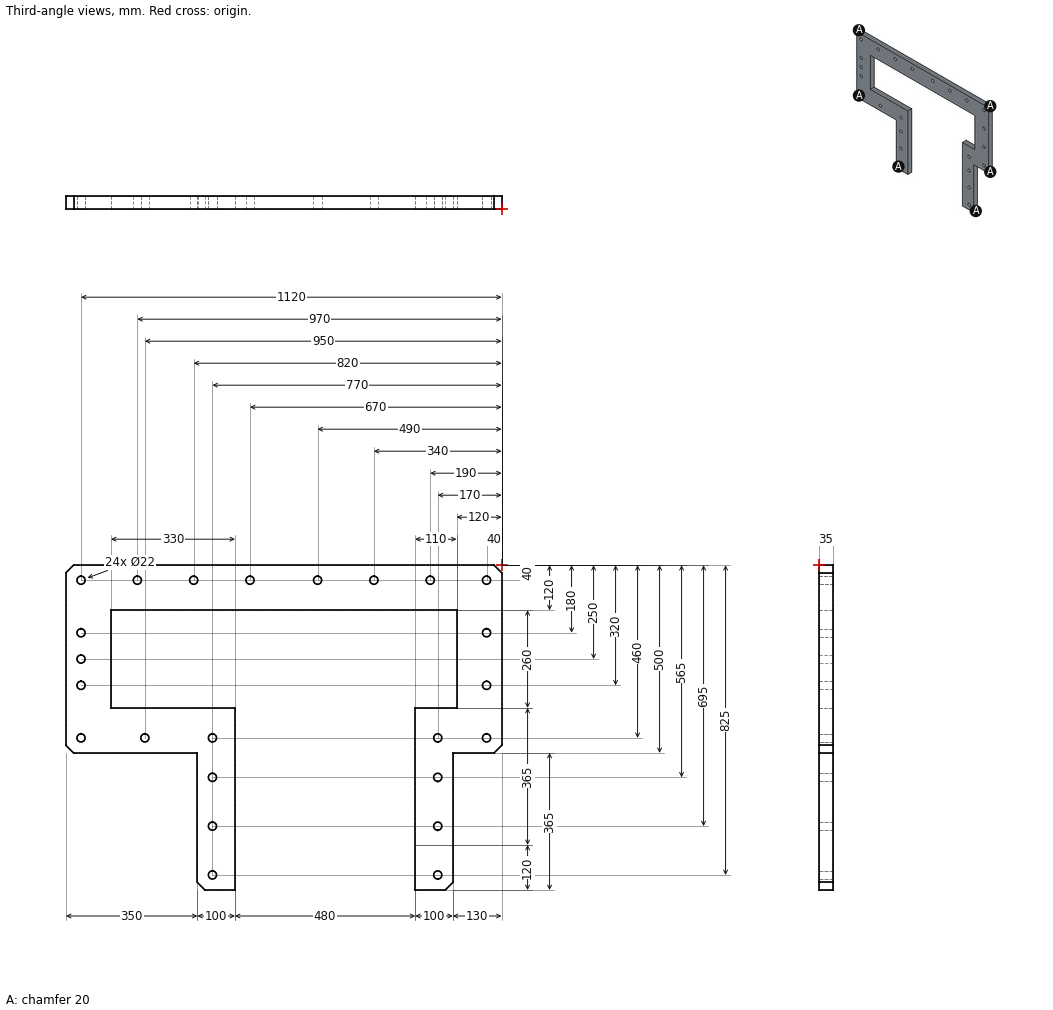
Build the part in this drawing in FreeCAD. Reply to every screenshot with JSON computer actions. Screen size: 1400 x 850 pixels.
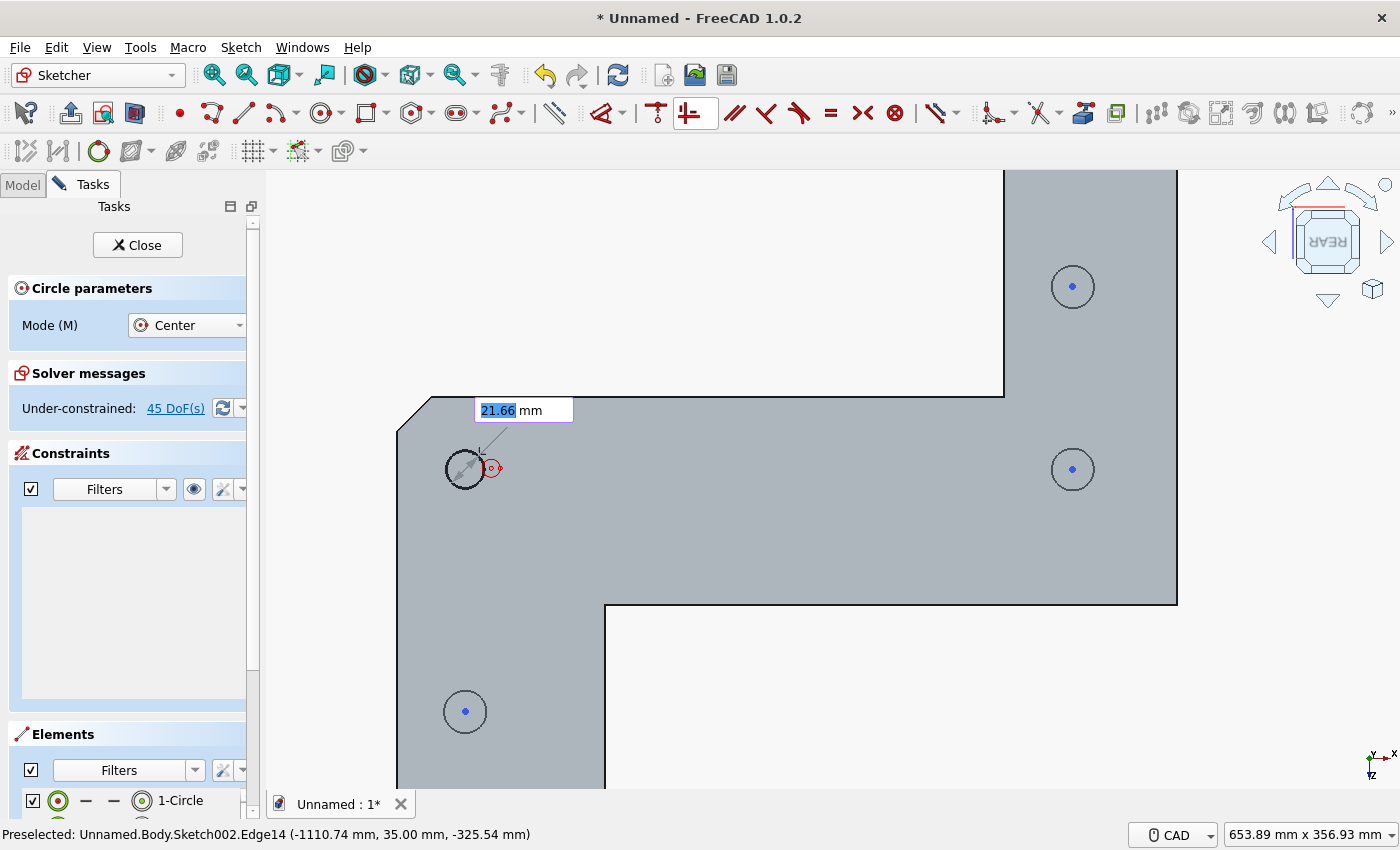
{"action": "left_click", "coordinate": [480, 453]}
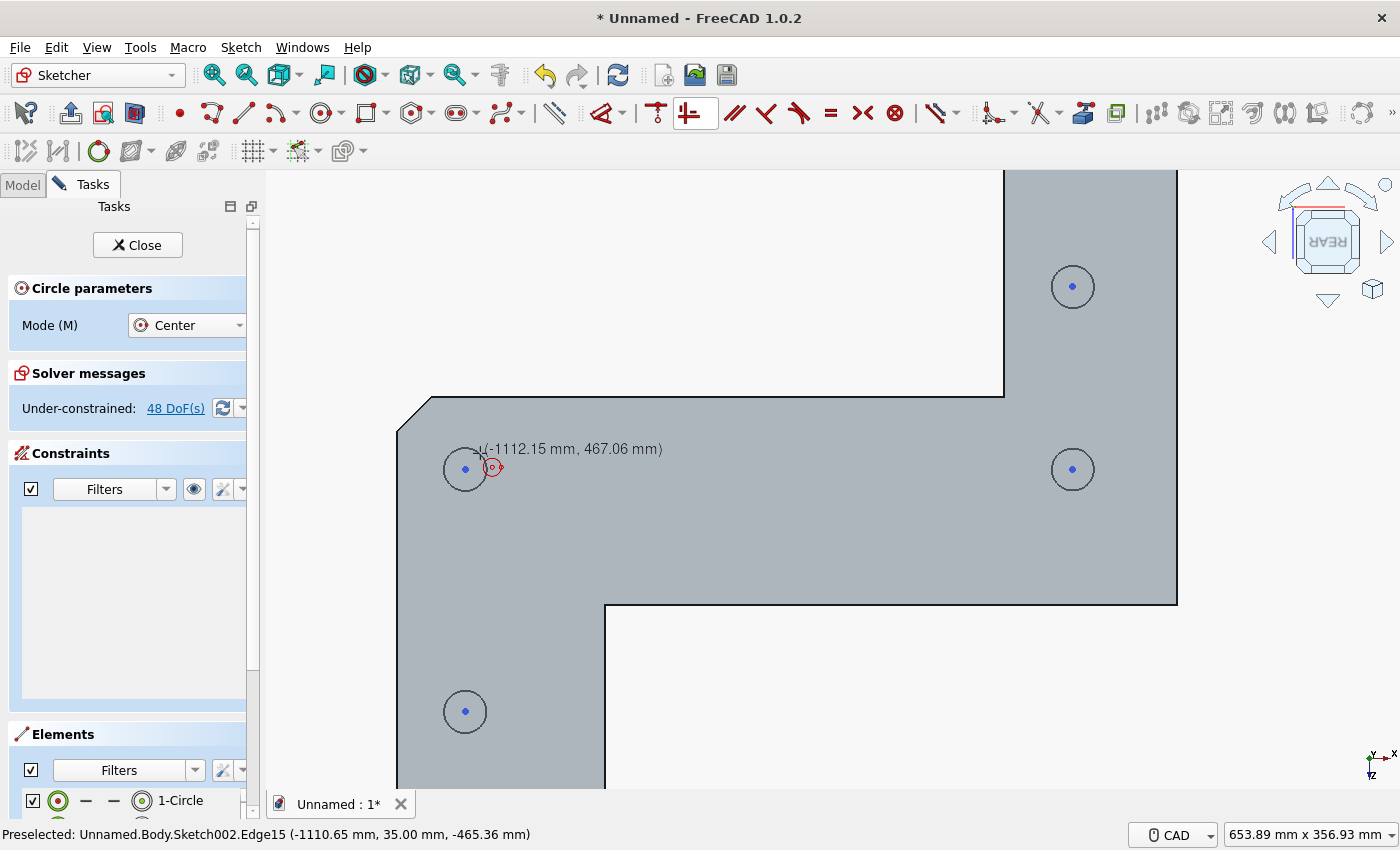
{"action": "scroll", "coordinate": [479, 454], "scroll_direction": "down", "scroll_amount": 6}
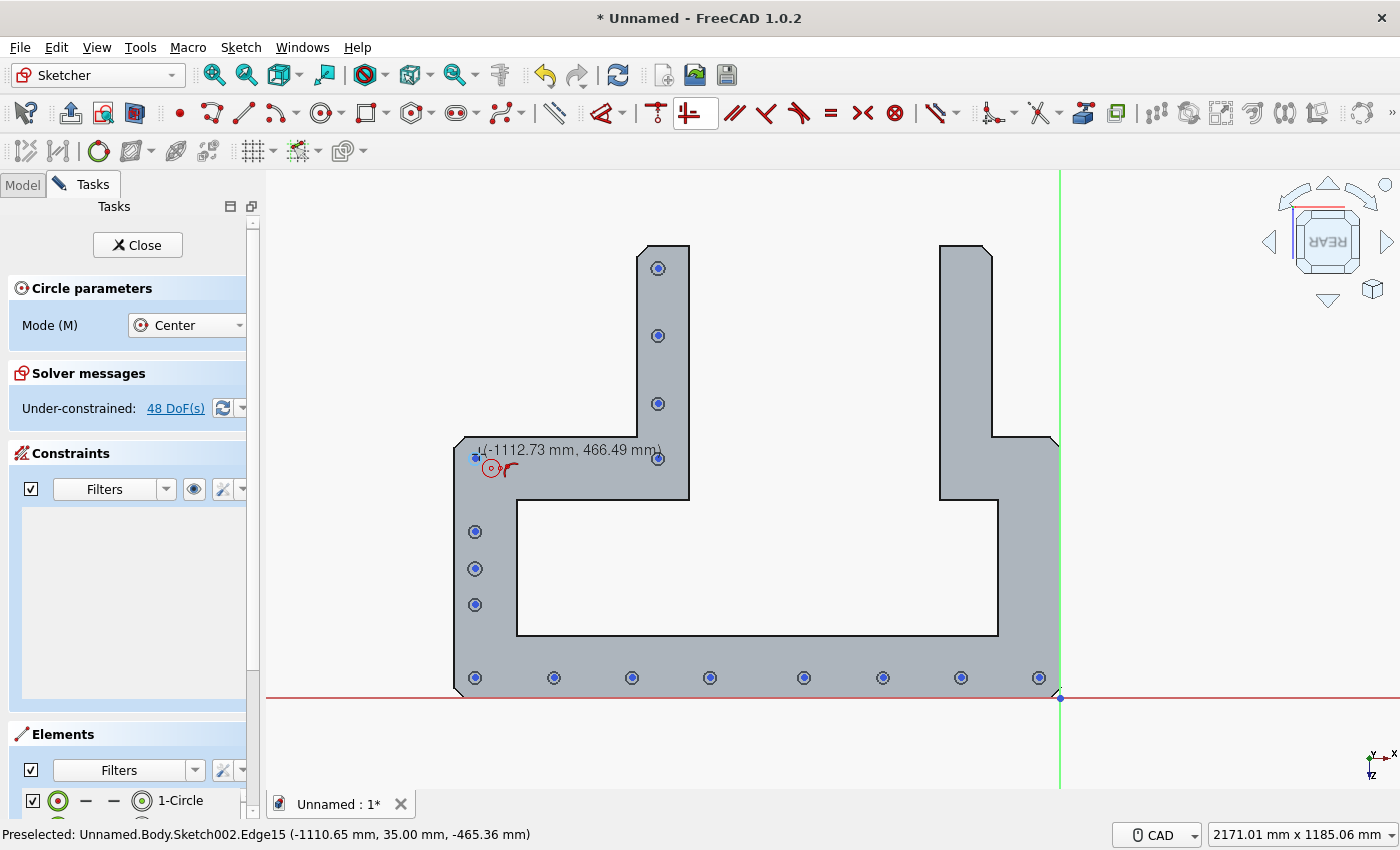
{"action": "left_click", "coordinate": [564, 458]}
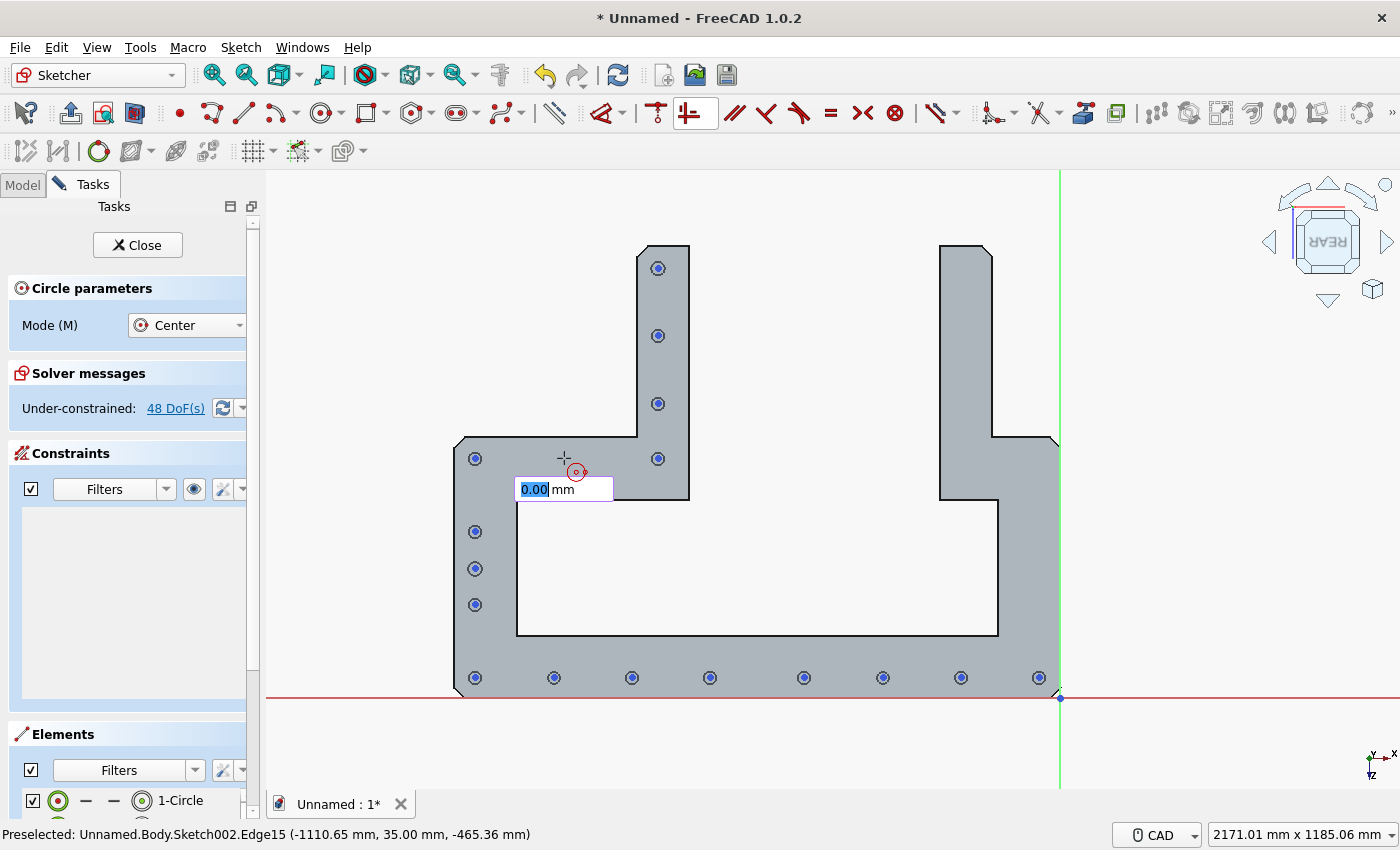
{"action": "scroll", "coordinate": [568, 454], "scroll_direction": "up", "scroll_amount": 6}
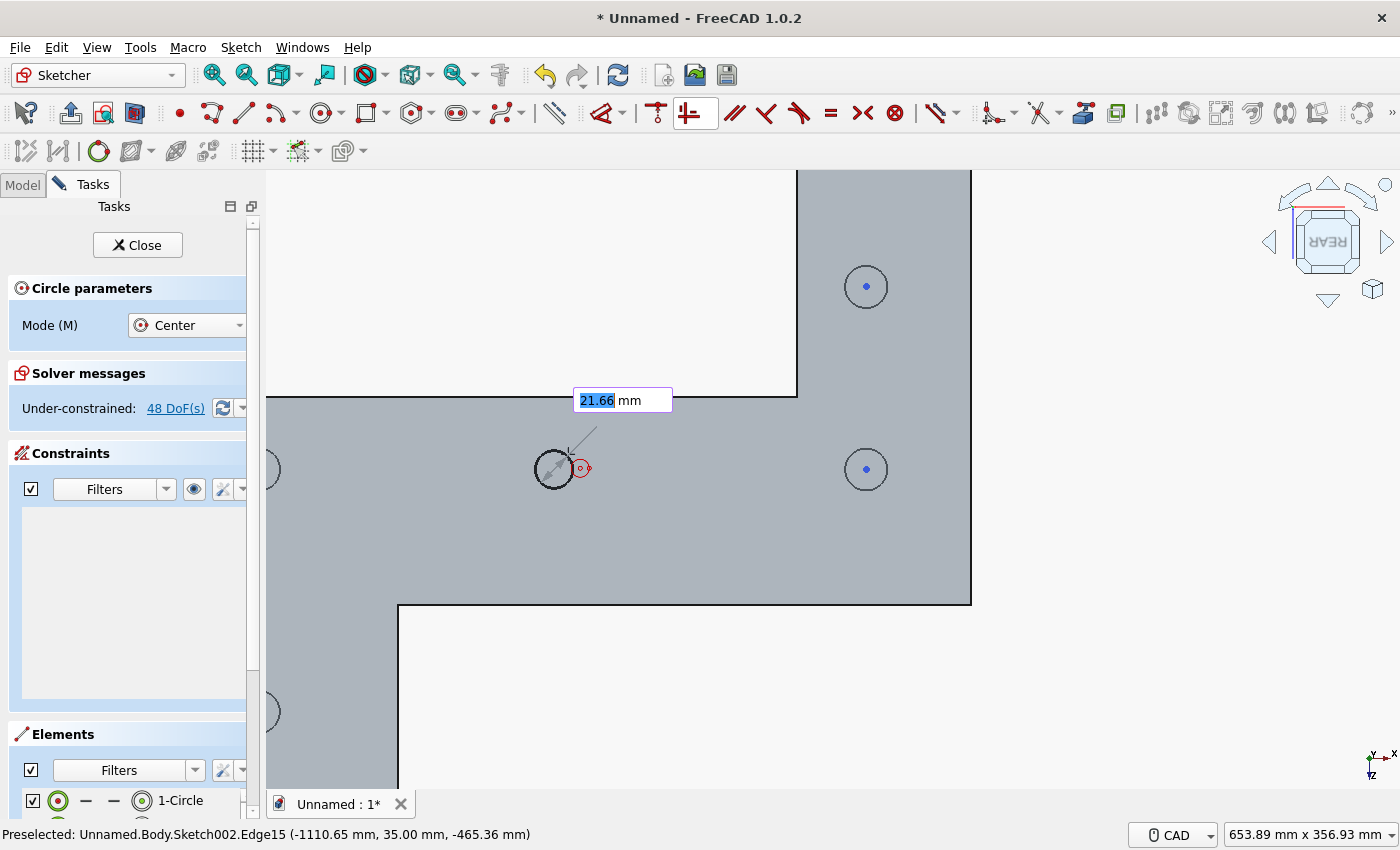
{"action": "left_click", "coordinate": [568, 453]}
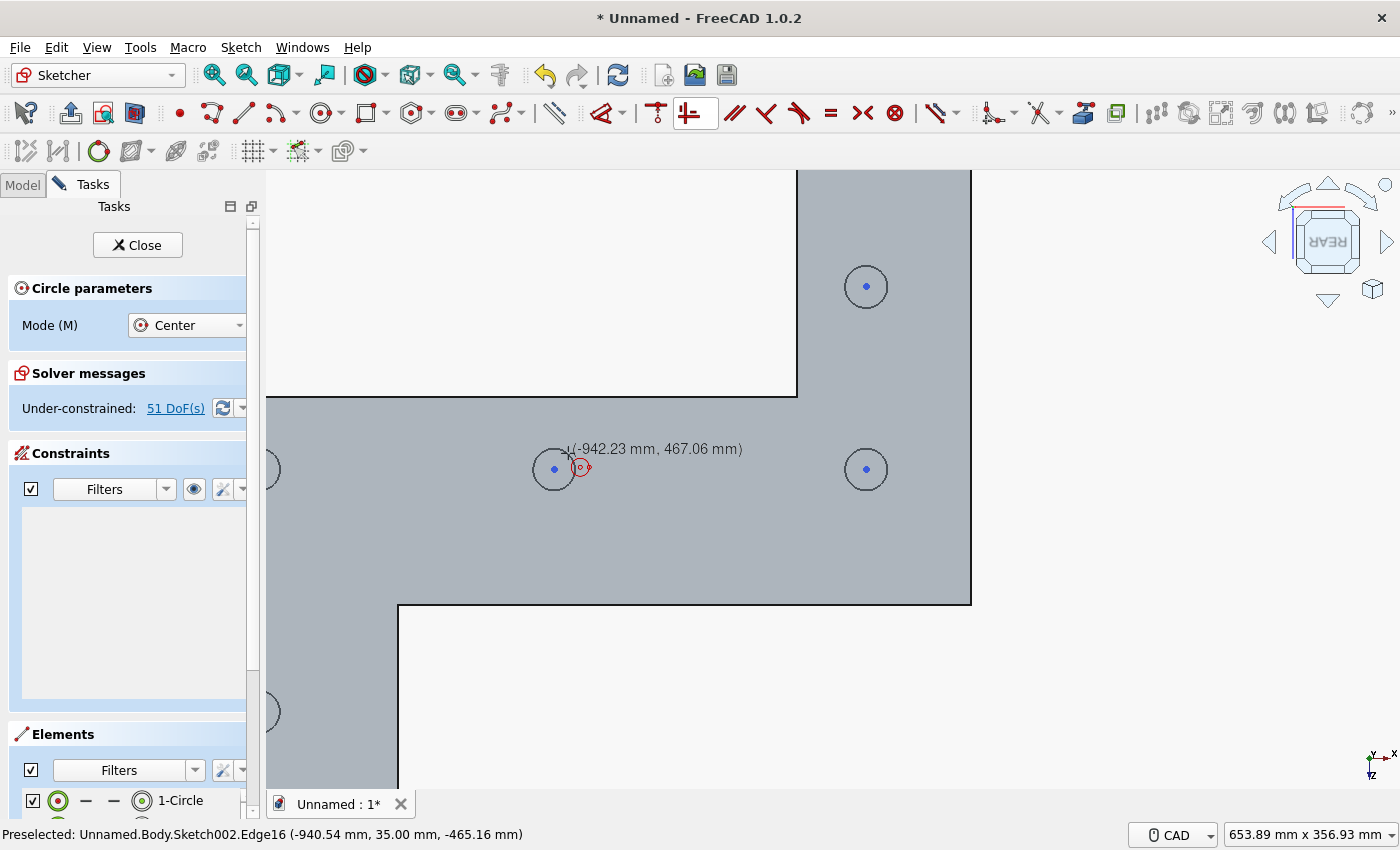
{"action": "scroll", "coordinate": [568, 454], "scroll_direction": "down", "scroll_amount": 6}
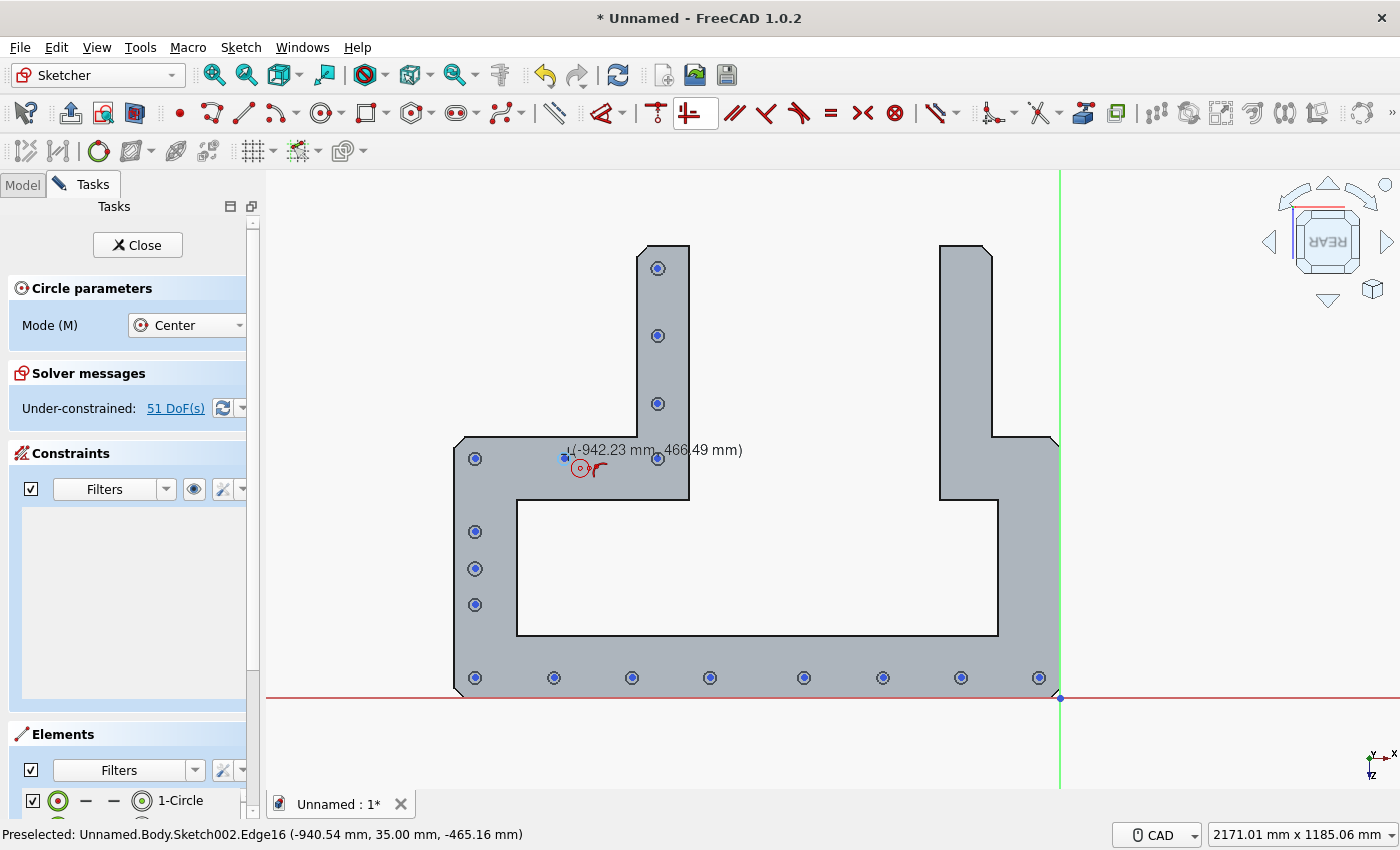
{"action": "scroll", "coordinate": [972, 458], "scroll_direction": "up", "scroll_amount": 7}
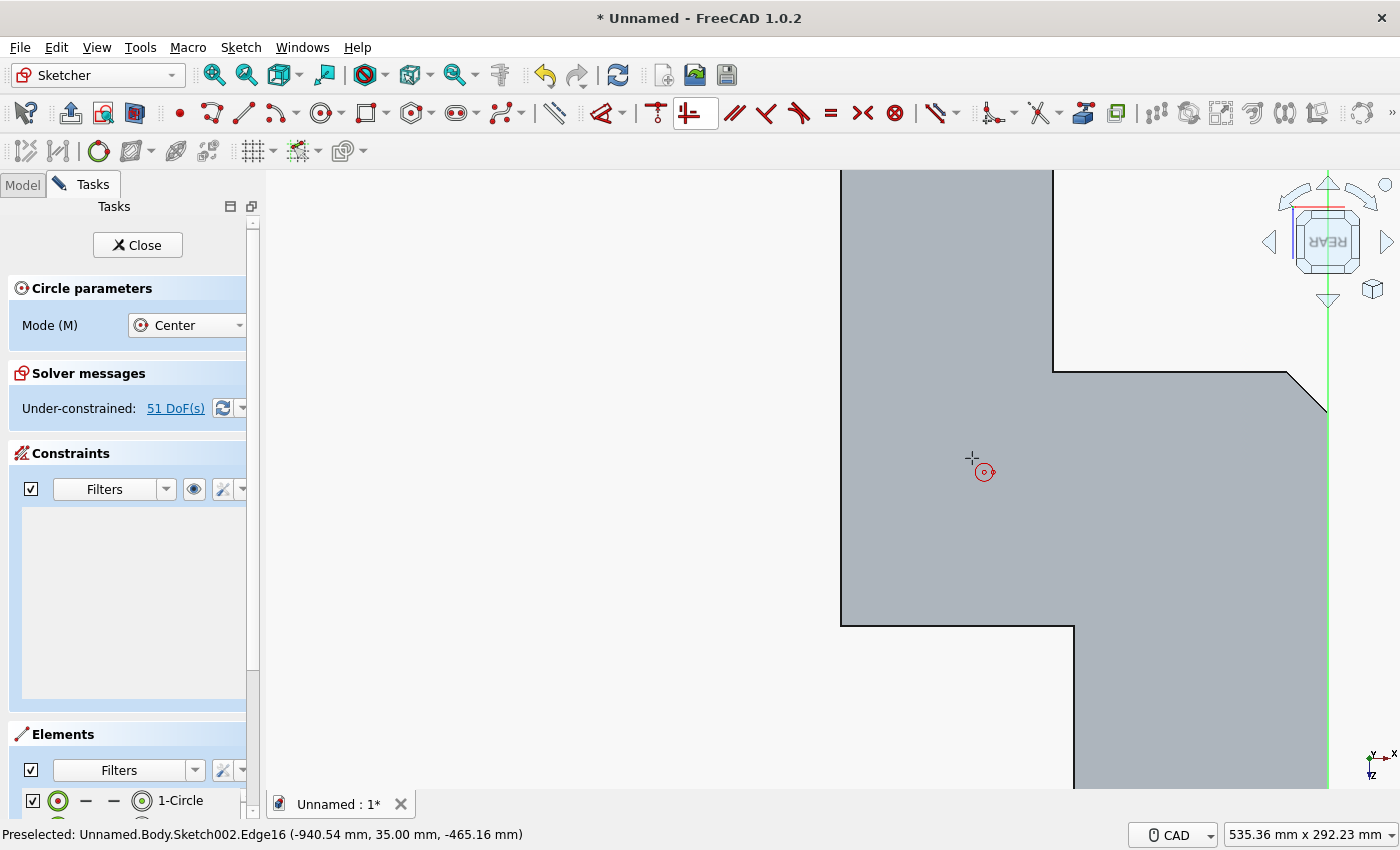
{"action": "scroll", "coordinate": [972, 458], "scroll_direction": "down", "scroll_amount": 7}